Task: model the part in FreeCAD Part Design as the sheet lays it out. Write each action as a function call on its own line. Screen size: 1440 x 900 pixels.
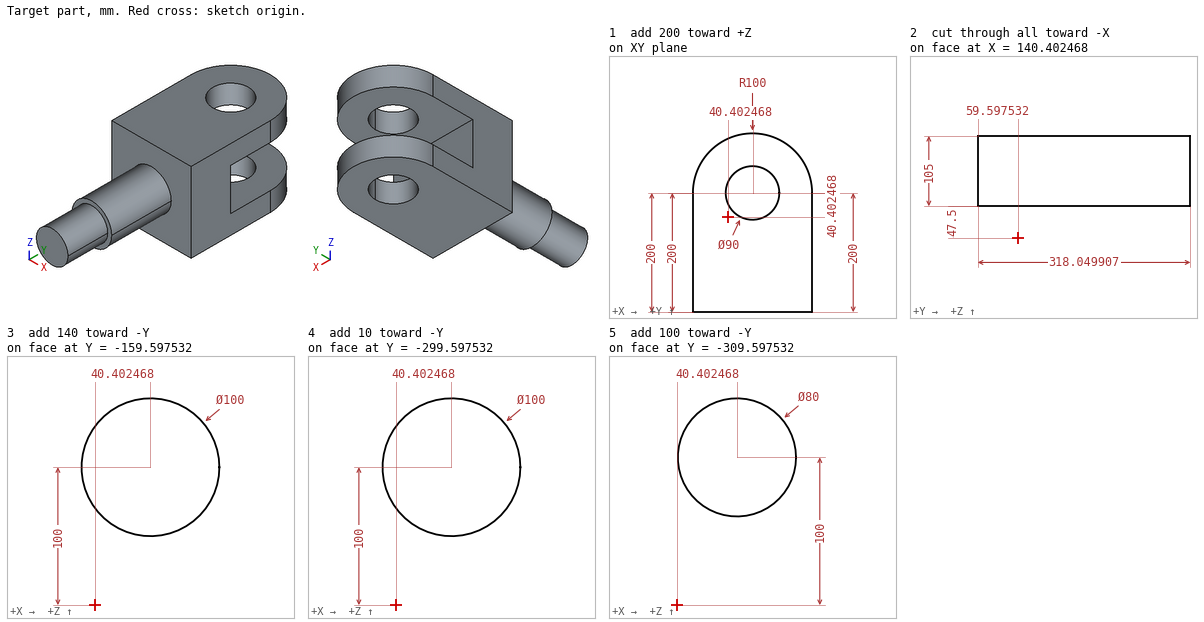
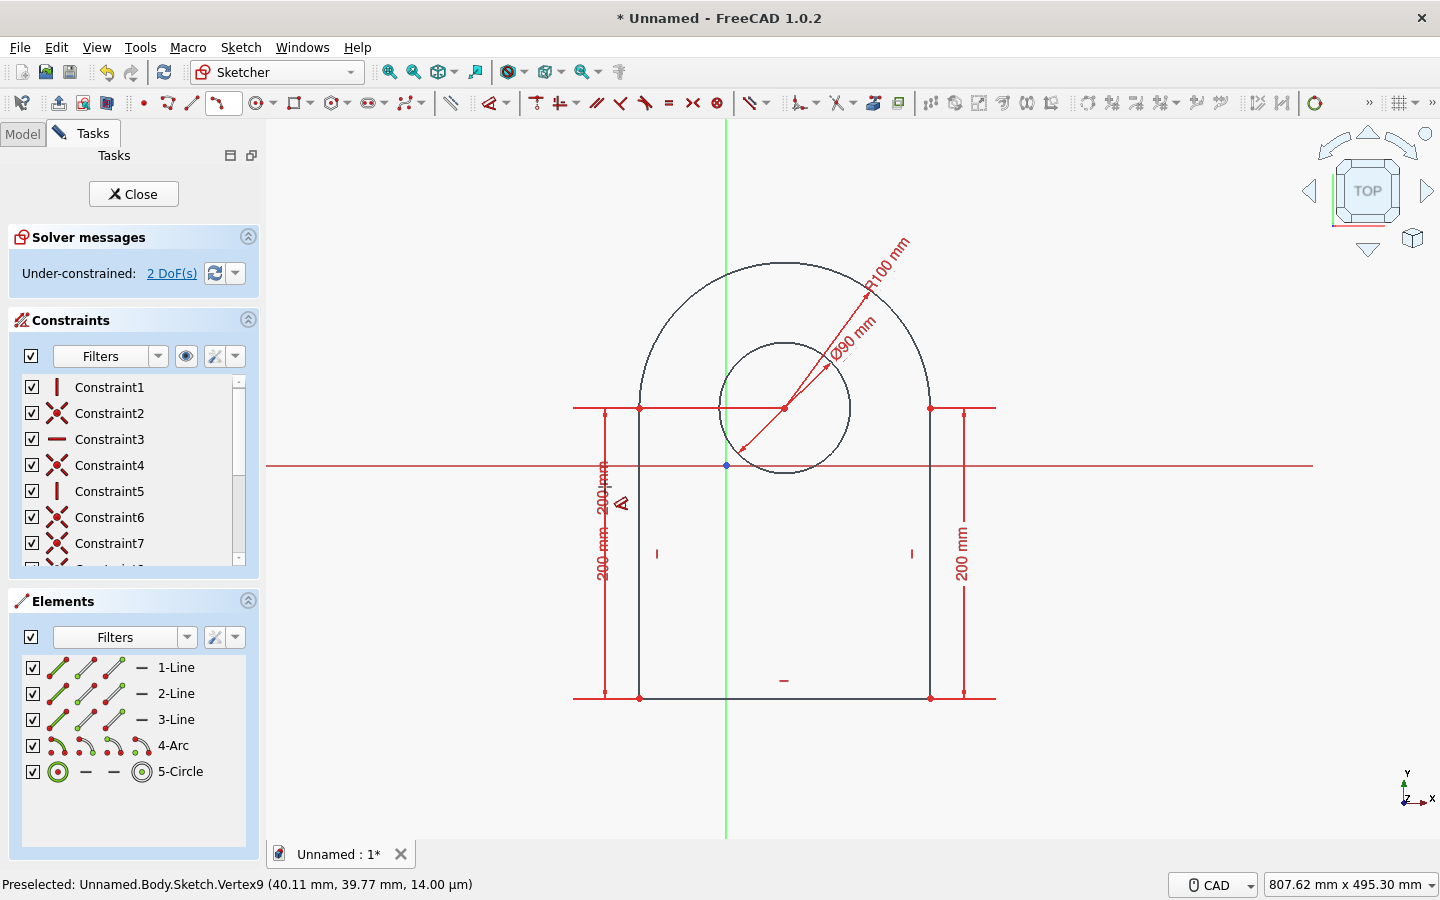
click(785, 408)
click(756, 374)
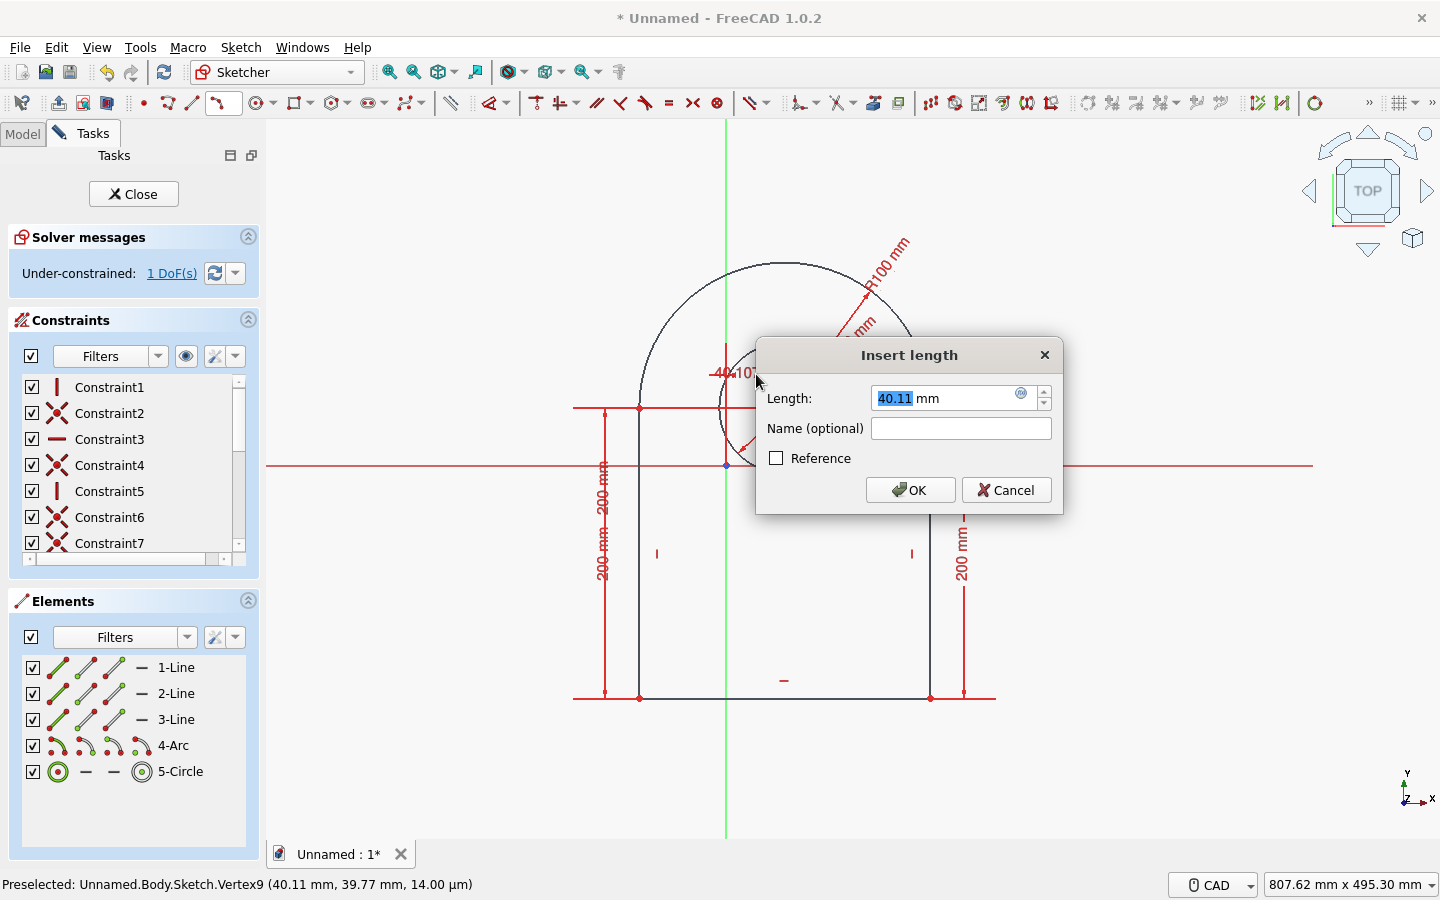
text(40.402468)
key(Return)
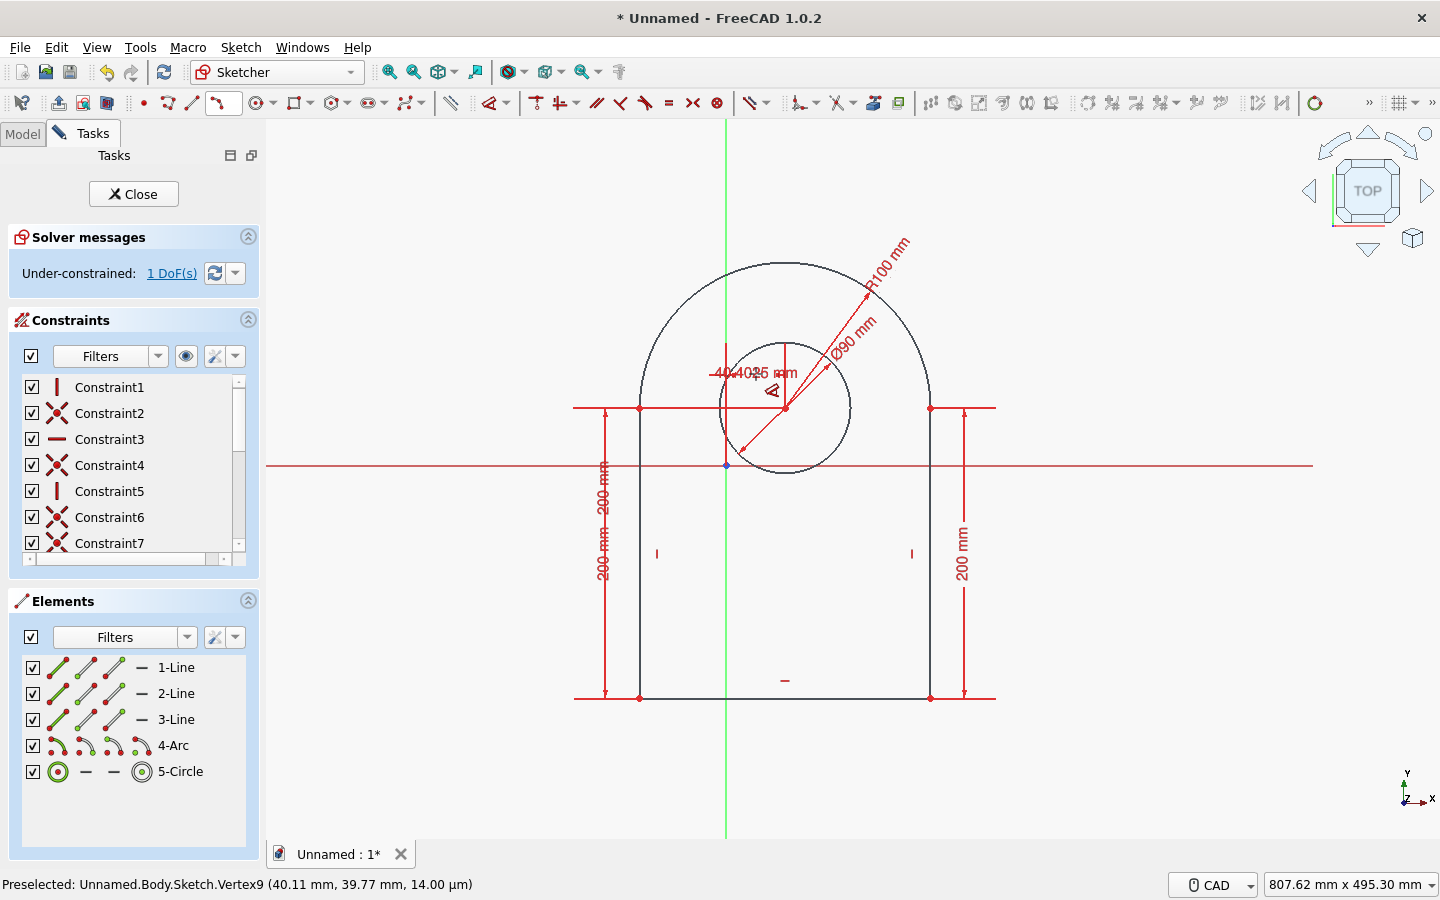
click(785, 408)
click(692, 437)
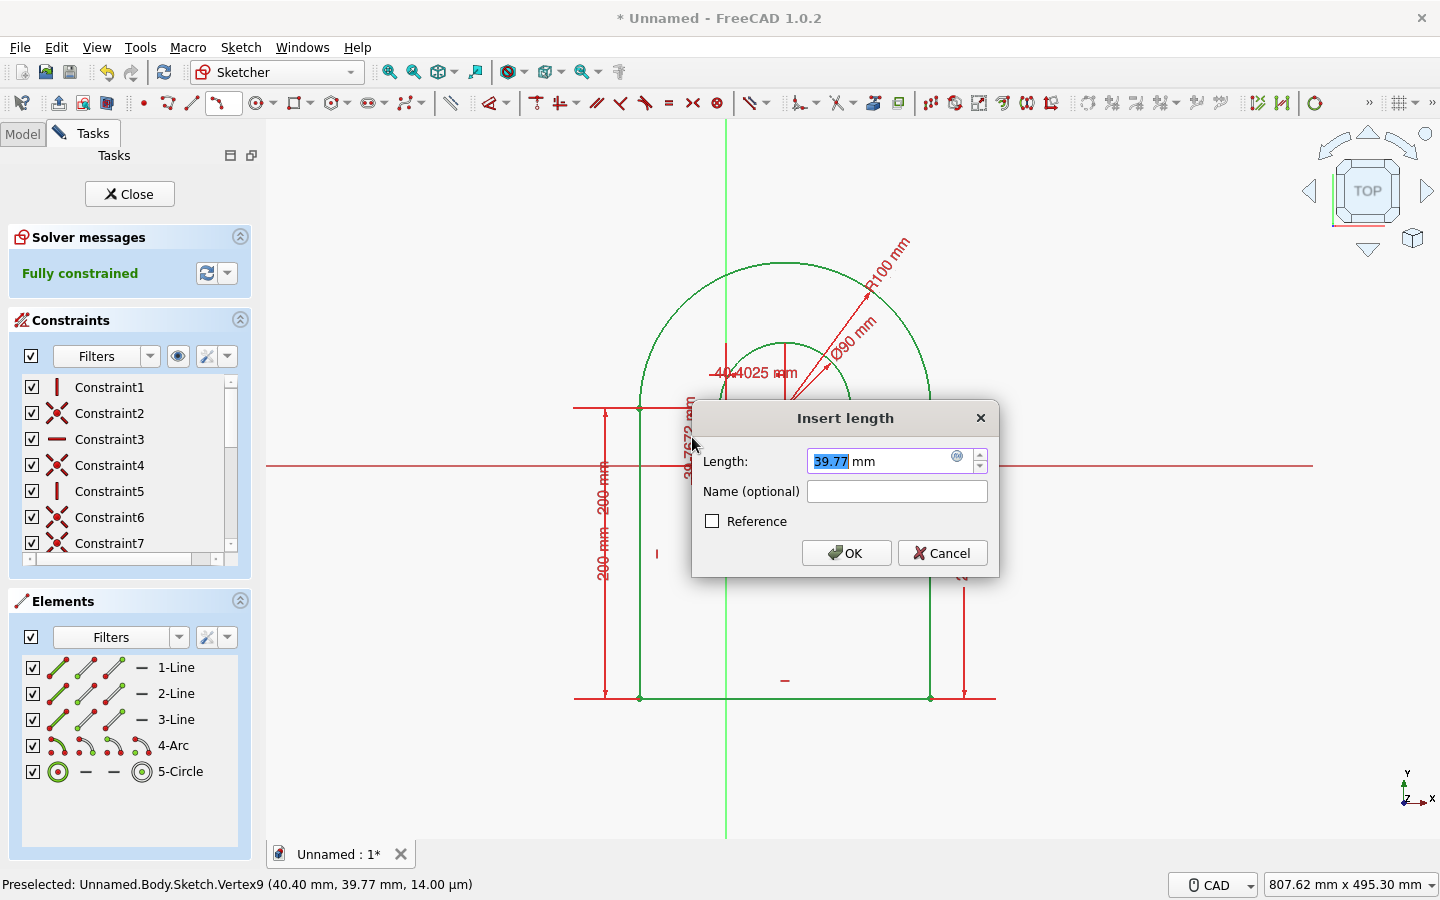
text(40.402468)
key(Return)
key(Escape)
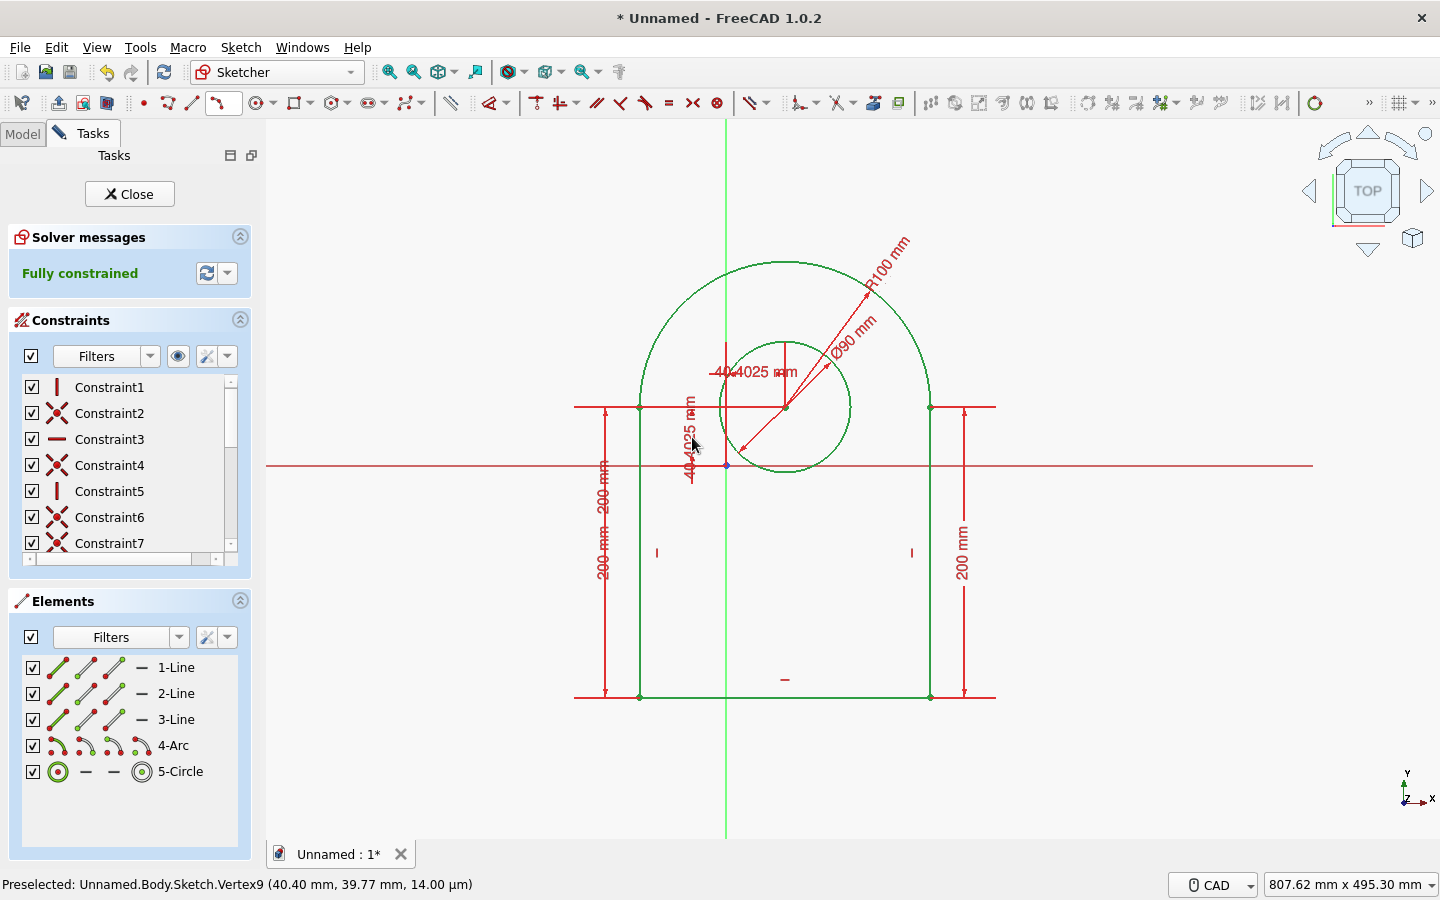
click(130, 194)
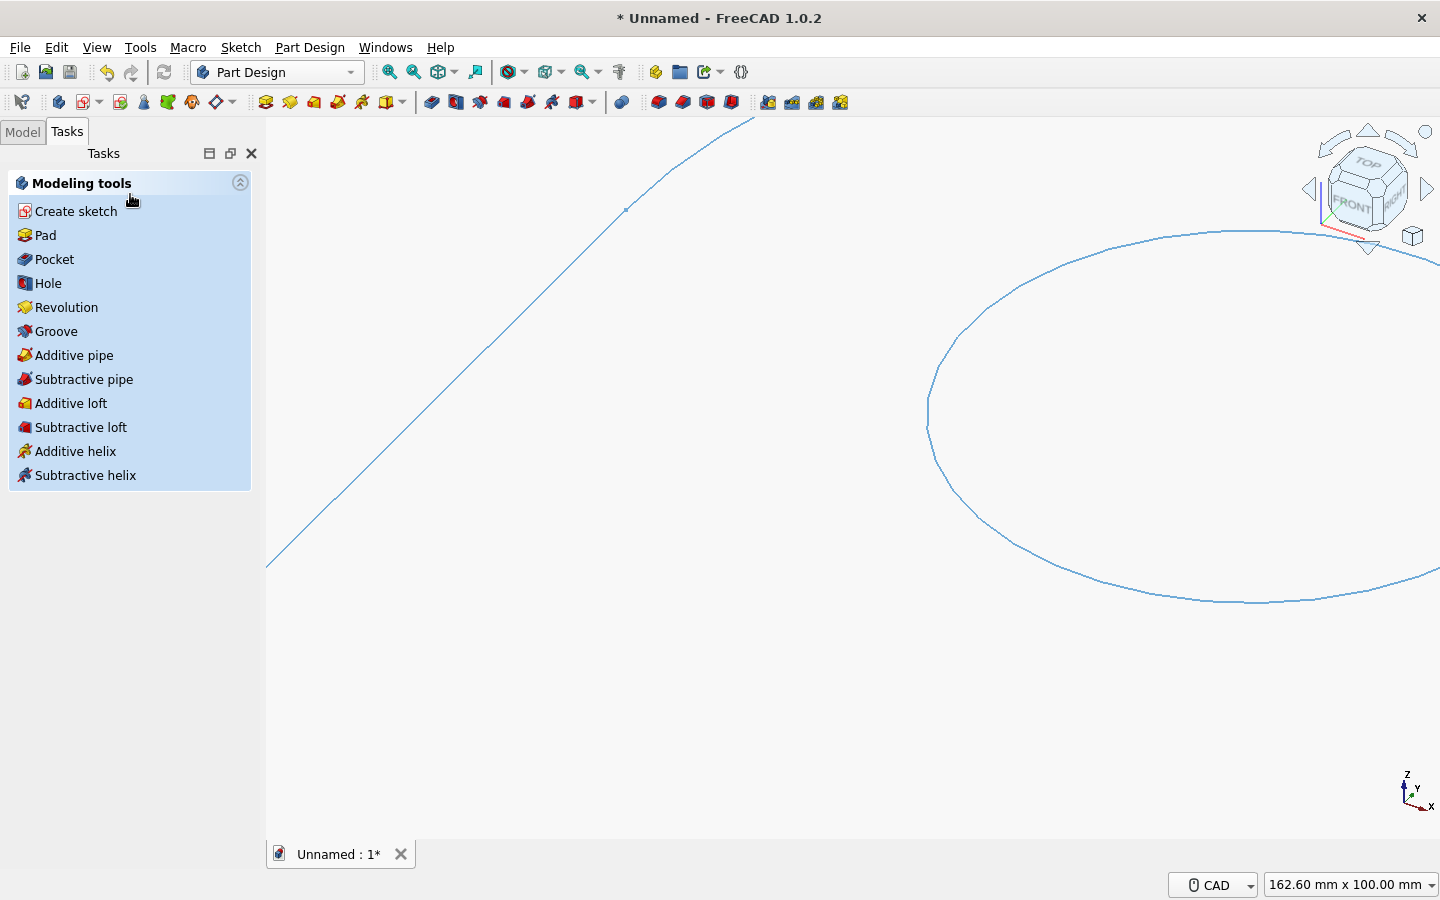
click(266, 102)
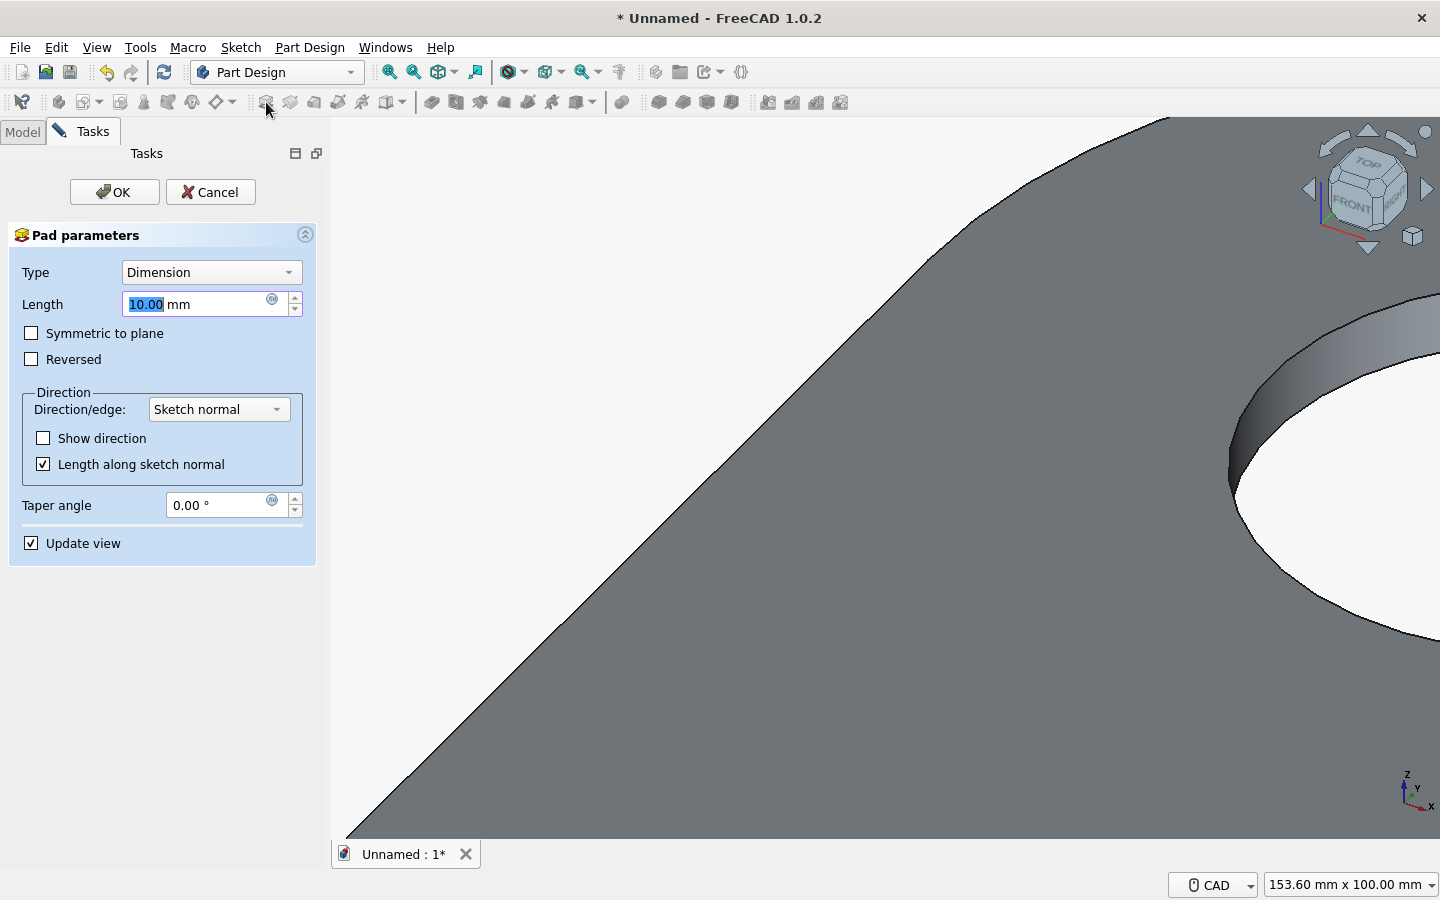
text(200)
key(Tab)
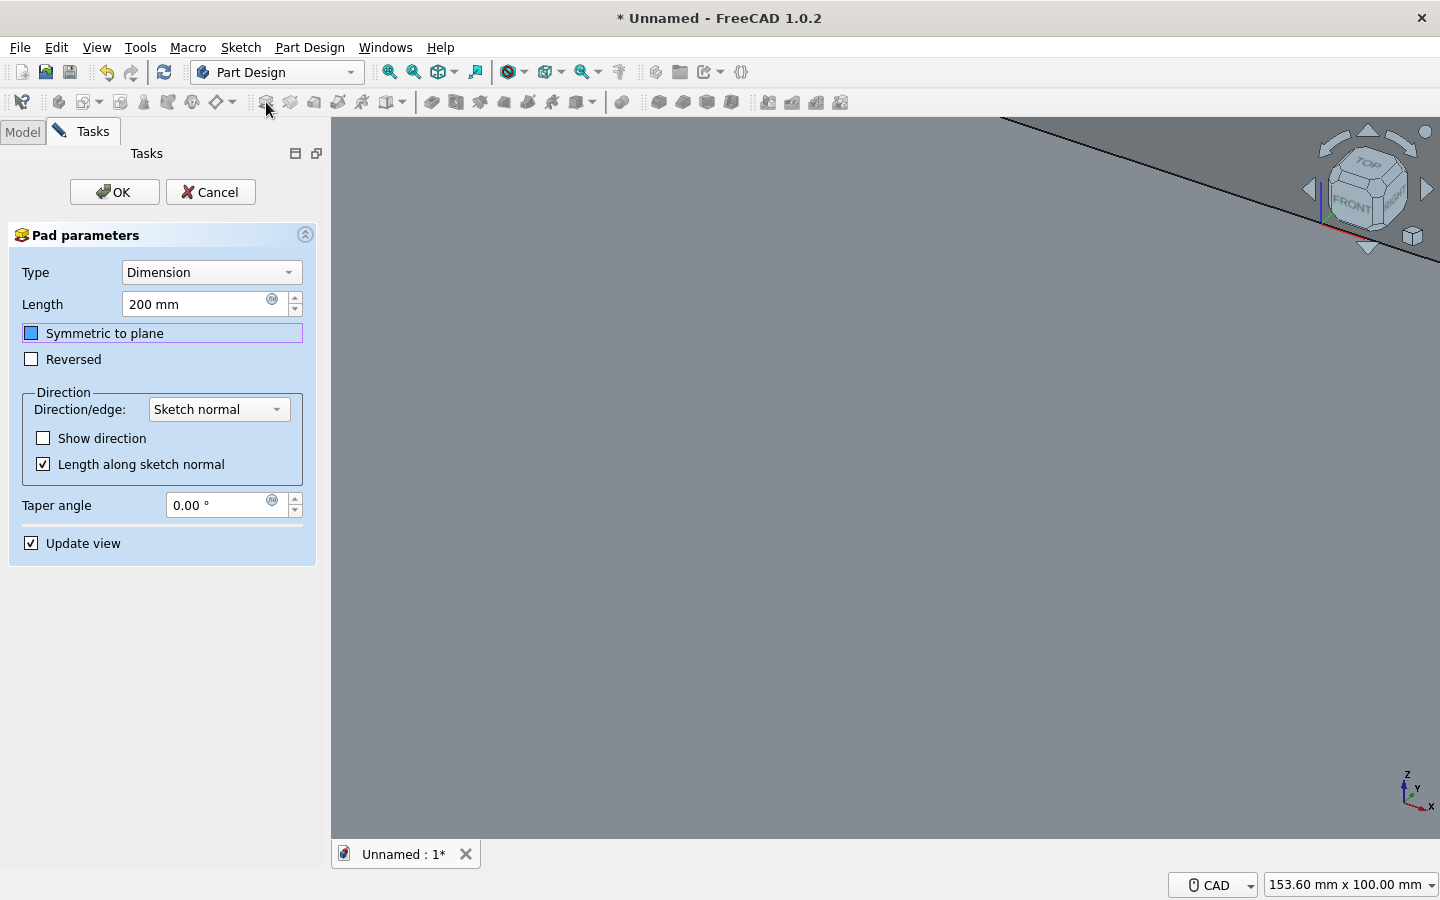
click(115, 192)